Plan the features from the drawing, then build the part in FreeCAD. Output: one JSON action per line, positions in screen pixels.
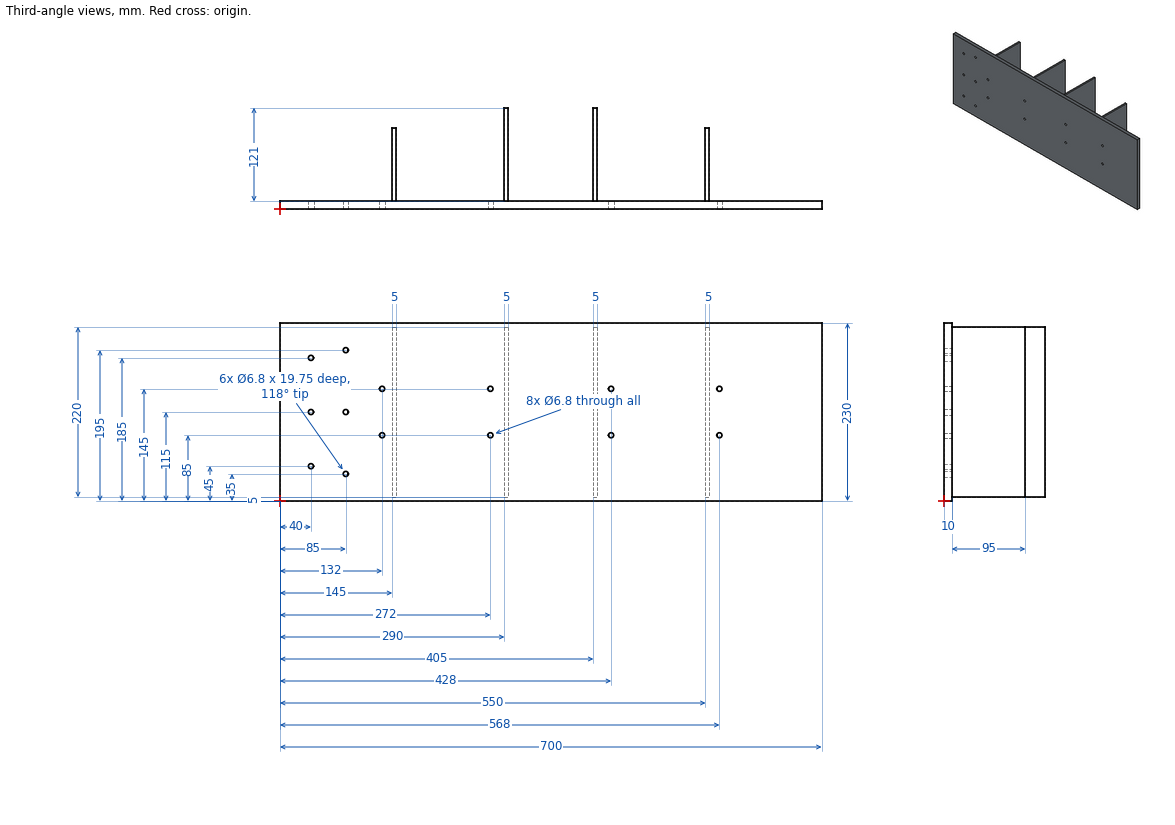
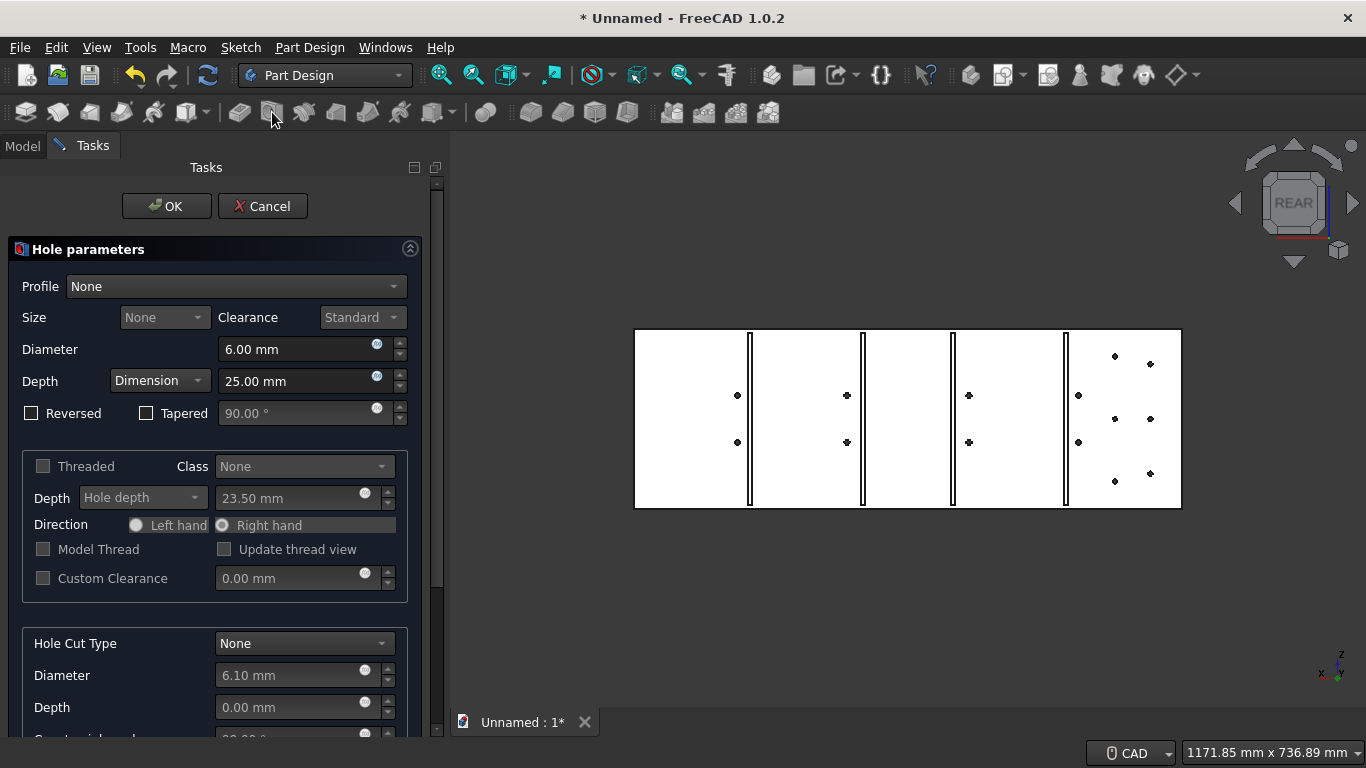
{"action": "triple_click", "coordinate": [305, 349]}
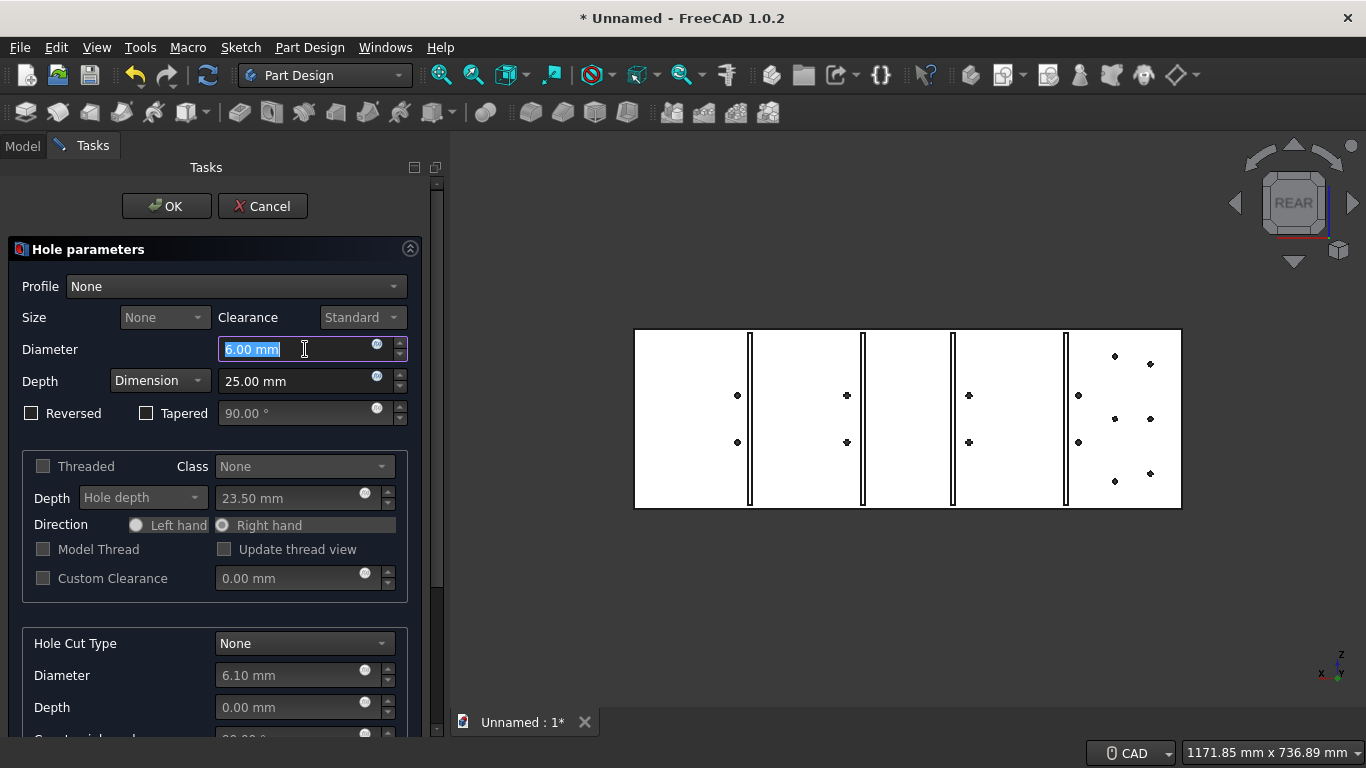
{"action": "type", "text": "6.8"}
{"action": "key", "text": "Tab"}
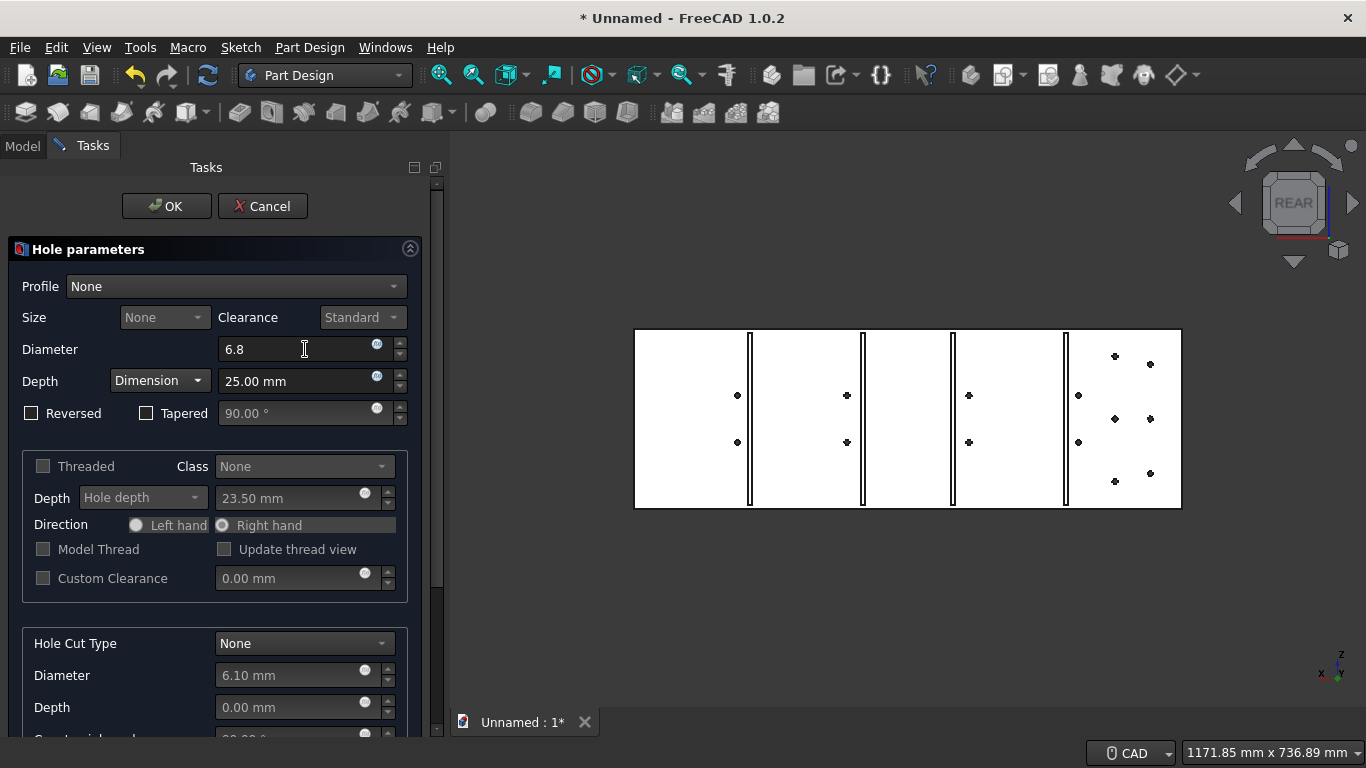
{"action": "triple_click", "coordinate": [305, 381]}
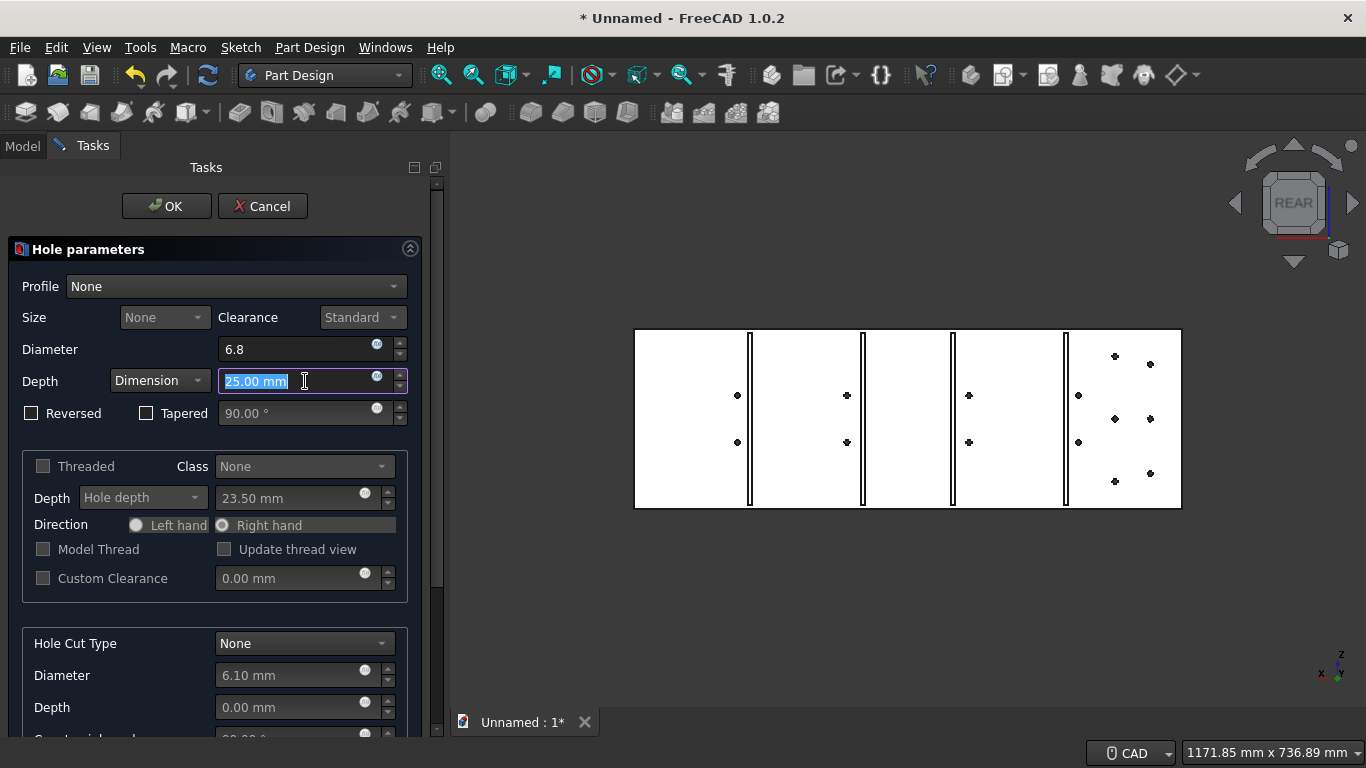
{"action": "type", "text": "19.75"}
{"action": "key", "text": "Tab"}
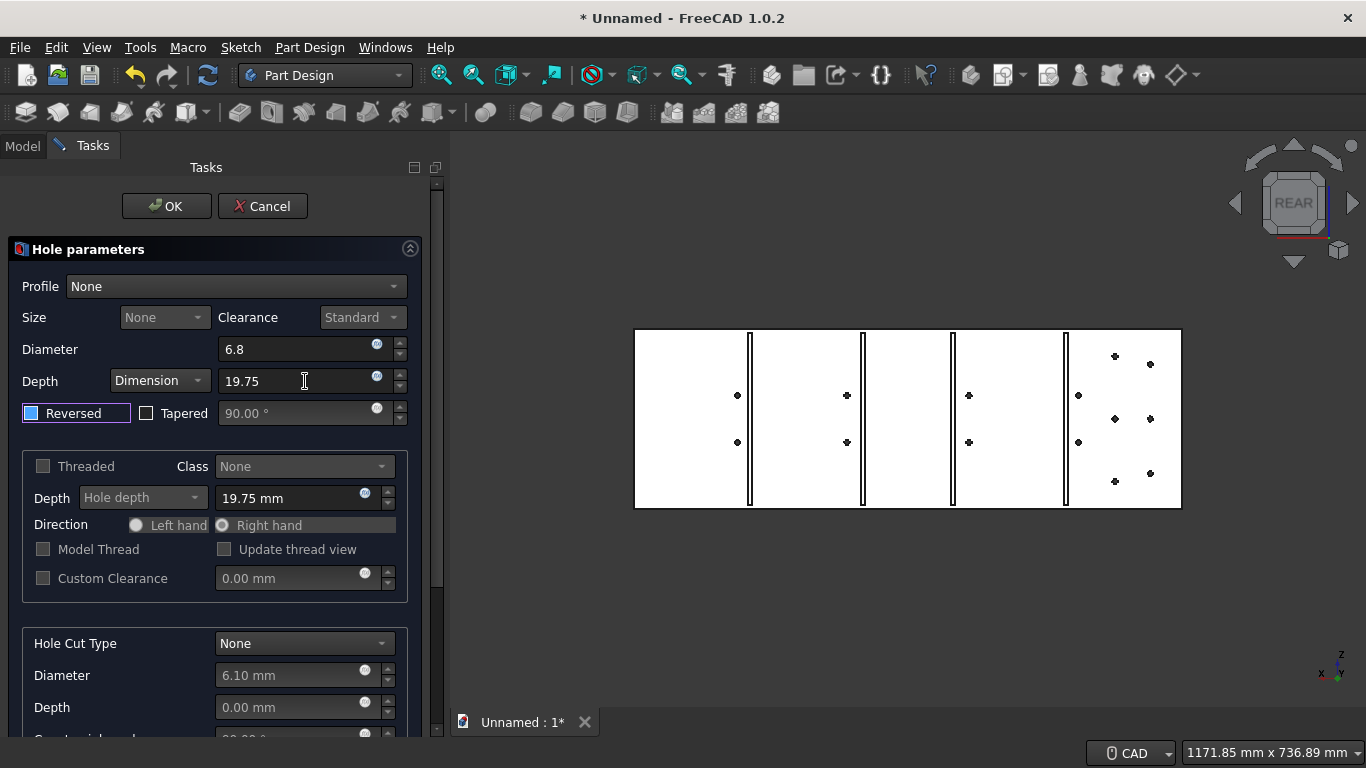
{"action": "left_click", "coordinate": [167, 206]}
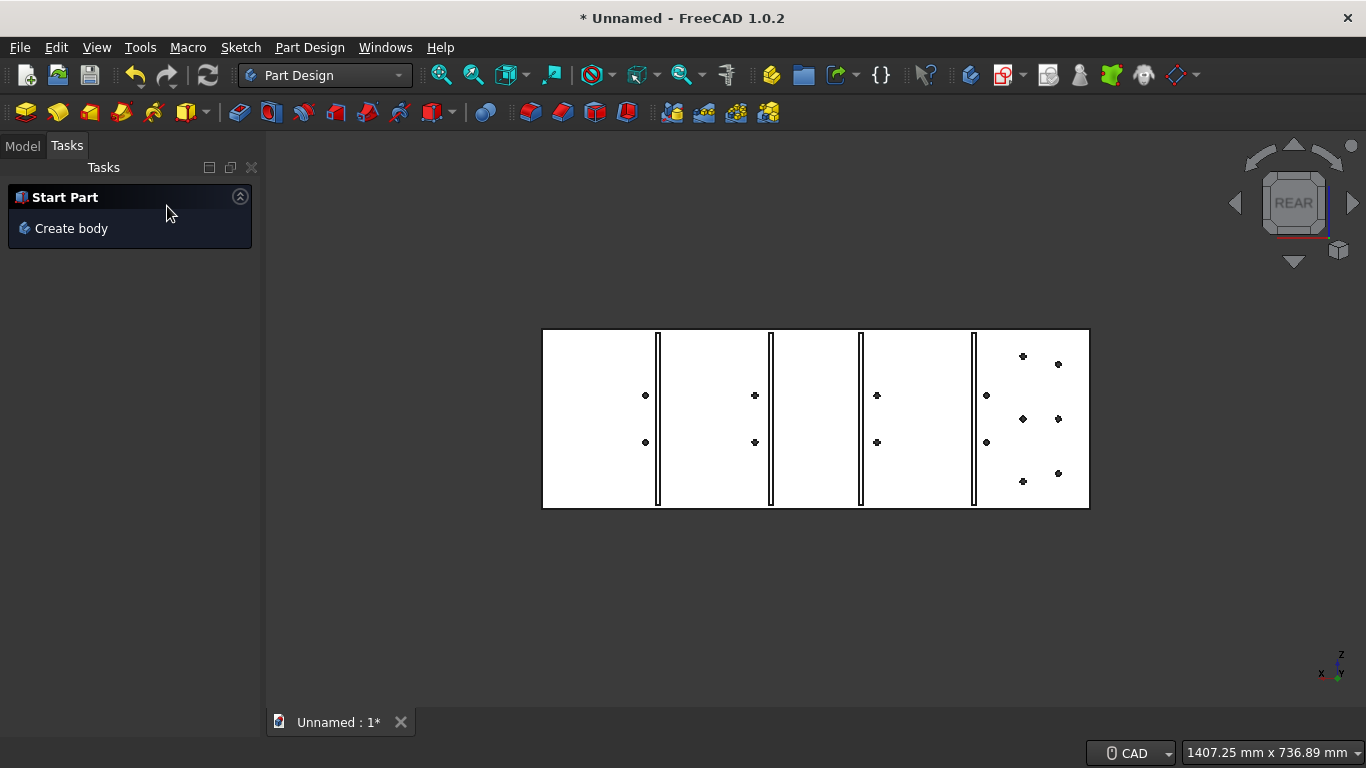
{"action": "key", "text": "0"}